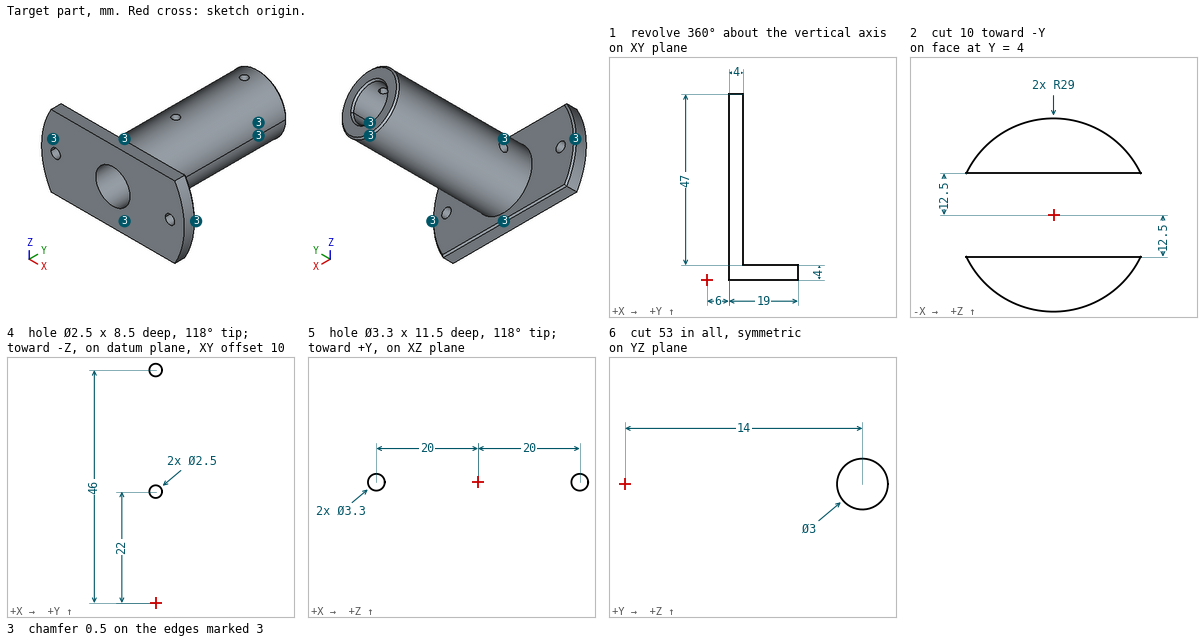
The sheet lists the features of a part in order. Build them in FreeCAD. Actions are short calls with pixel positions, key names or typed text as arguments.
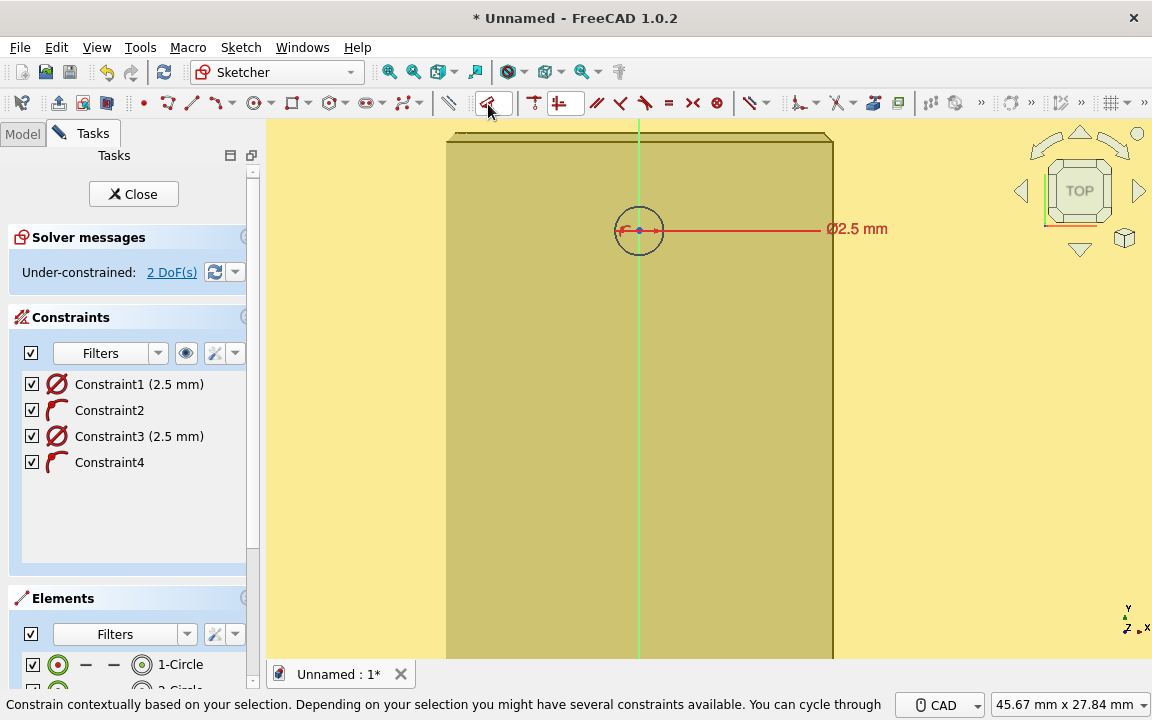
scroll(641, 229, down, 5)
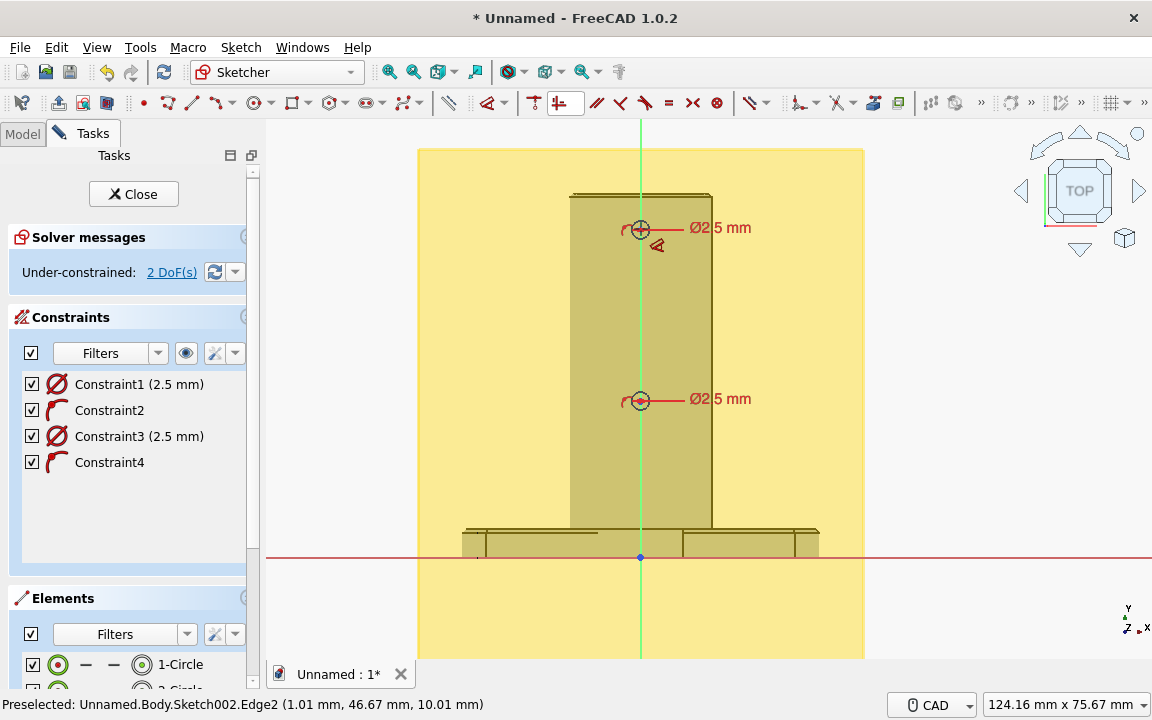
click(641, 401)
click(675, 479)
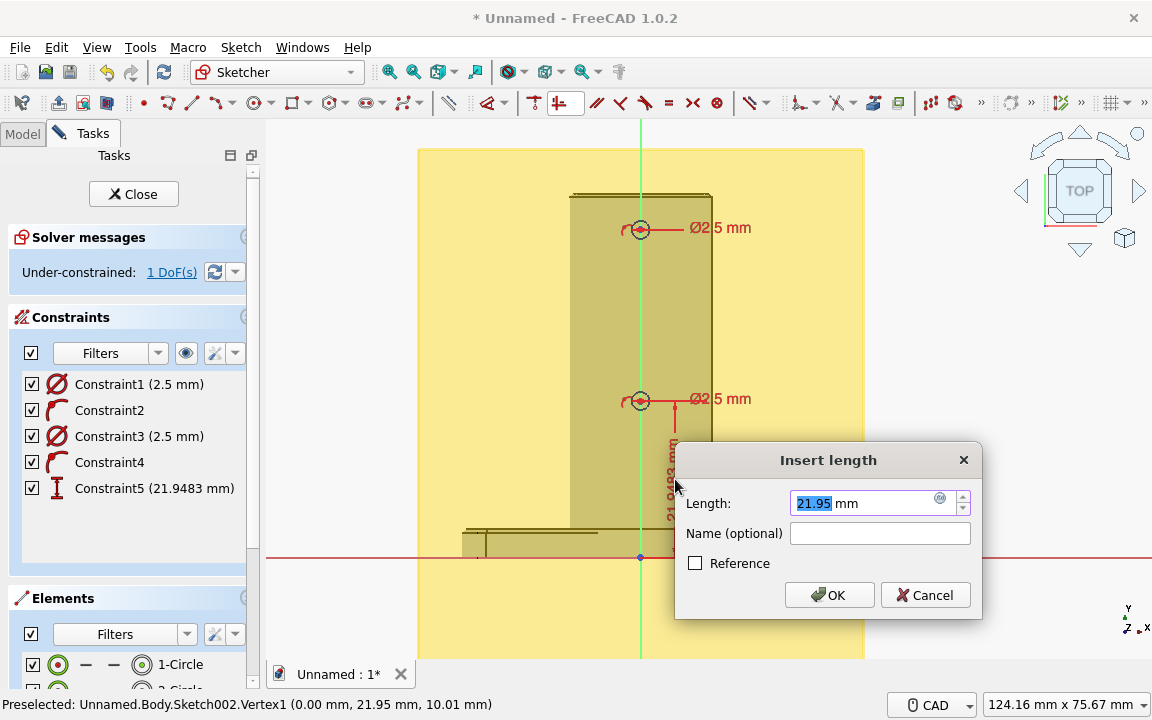
text(22)
key(Return)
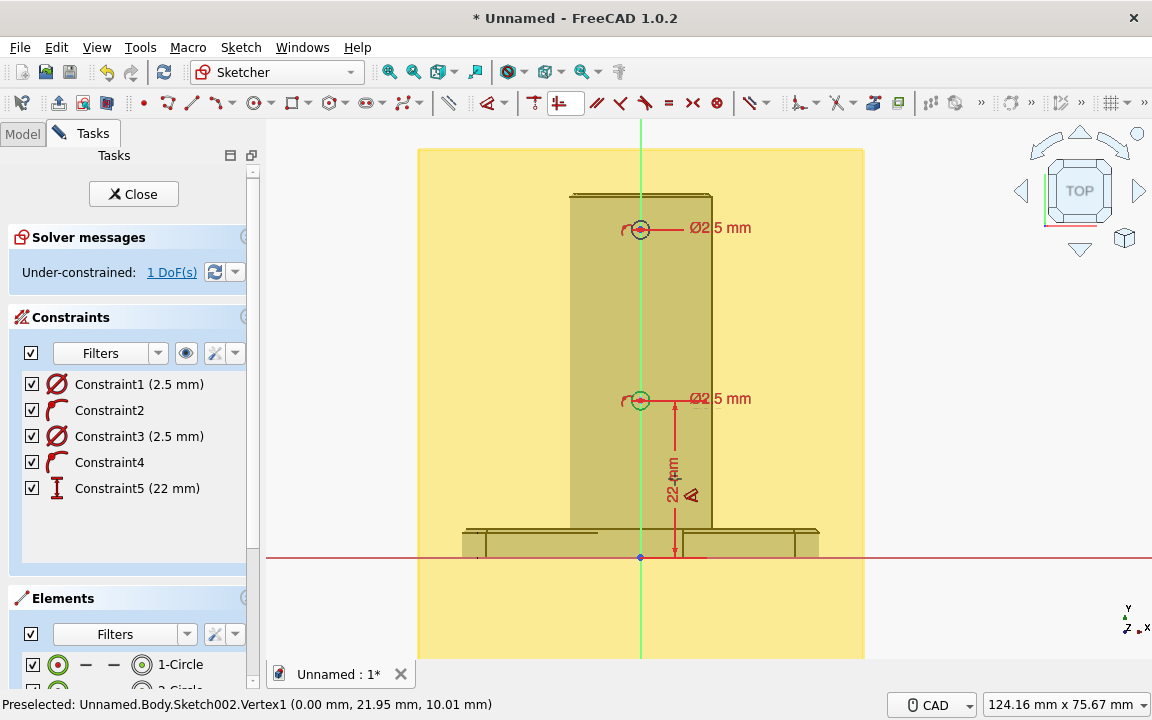
click(641, 230)
click(675, 394)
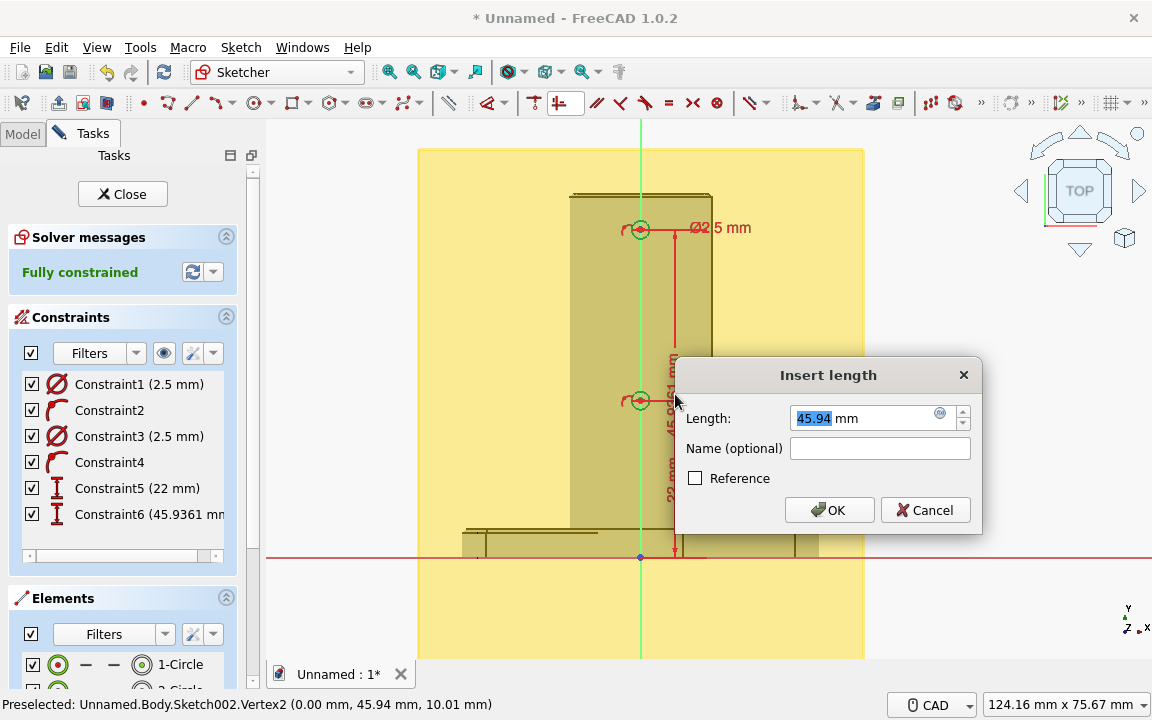
text(46)
key(Return)
key(Escape)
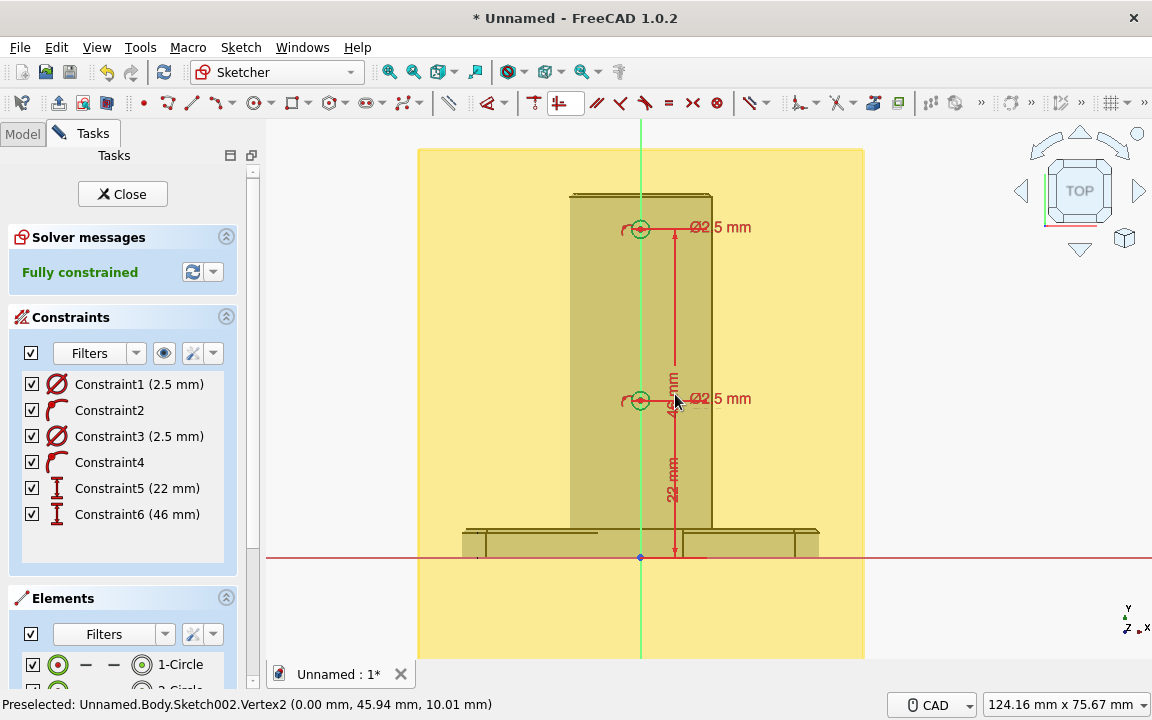
click(123, 194)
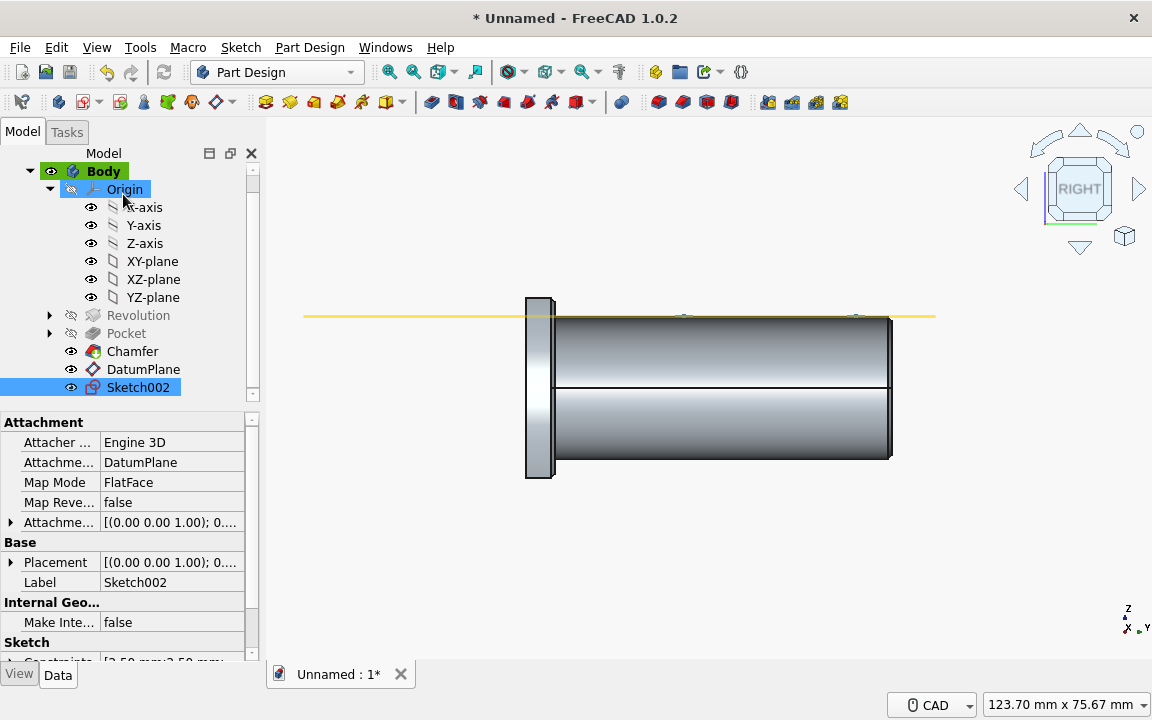
click(456, 102)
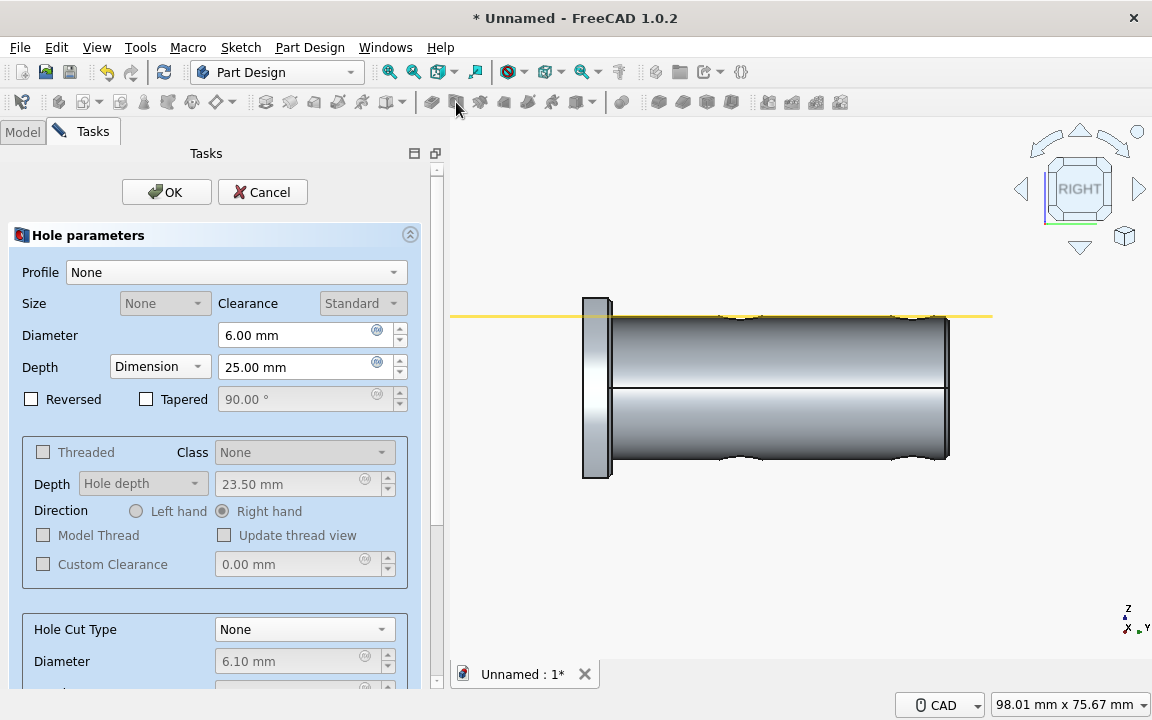
triple_click(305, 335)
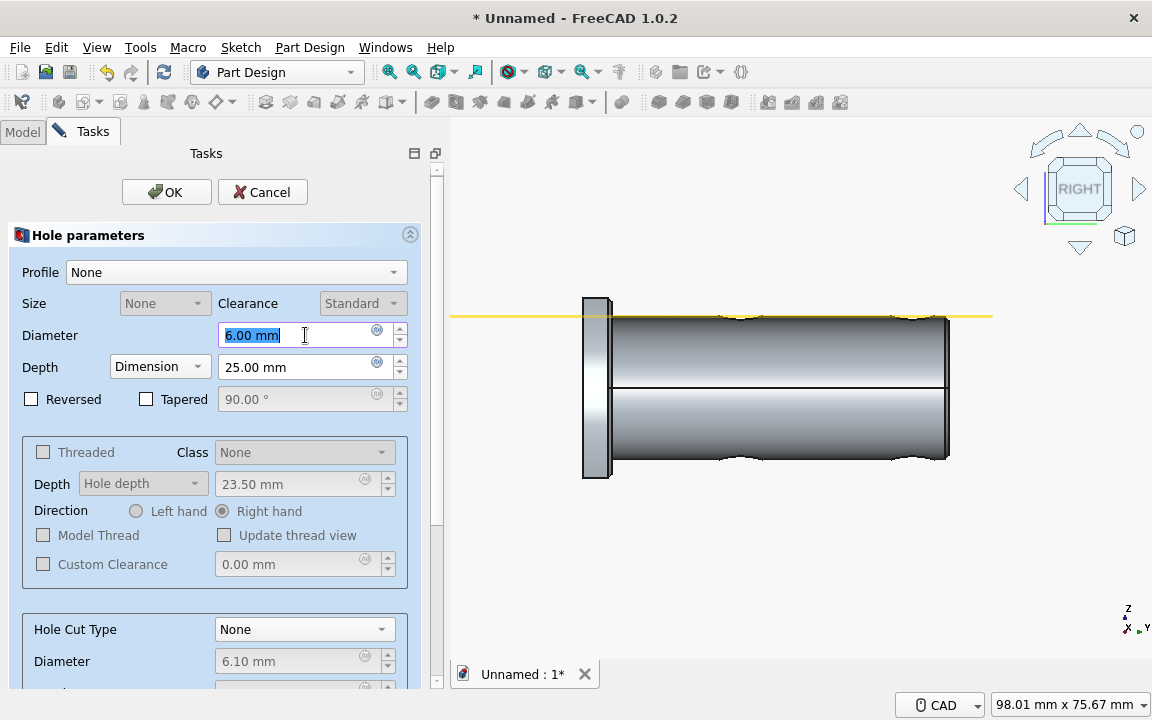
text(2.5)
key(Tab)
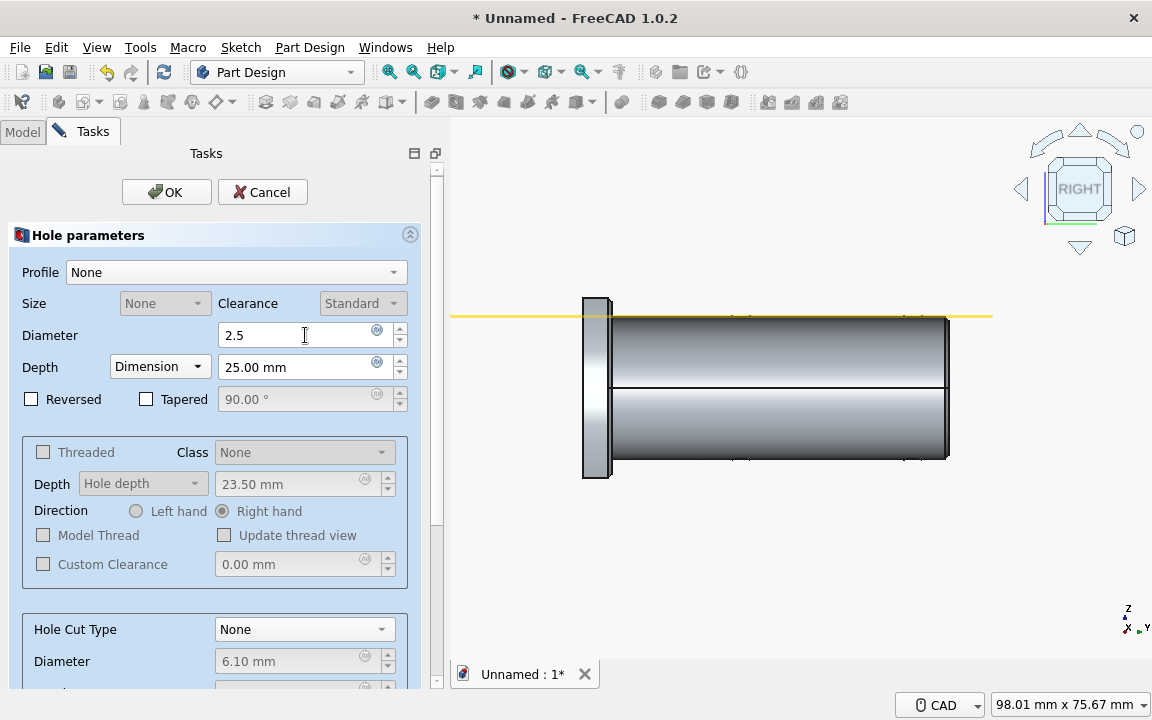
triple_click(305, 367)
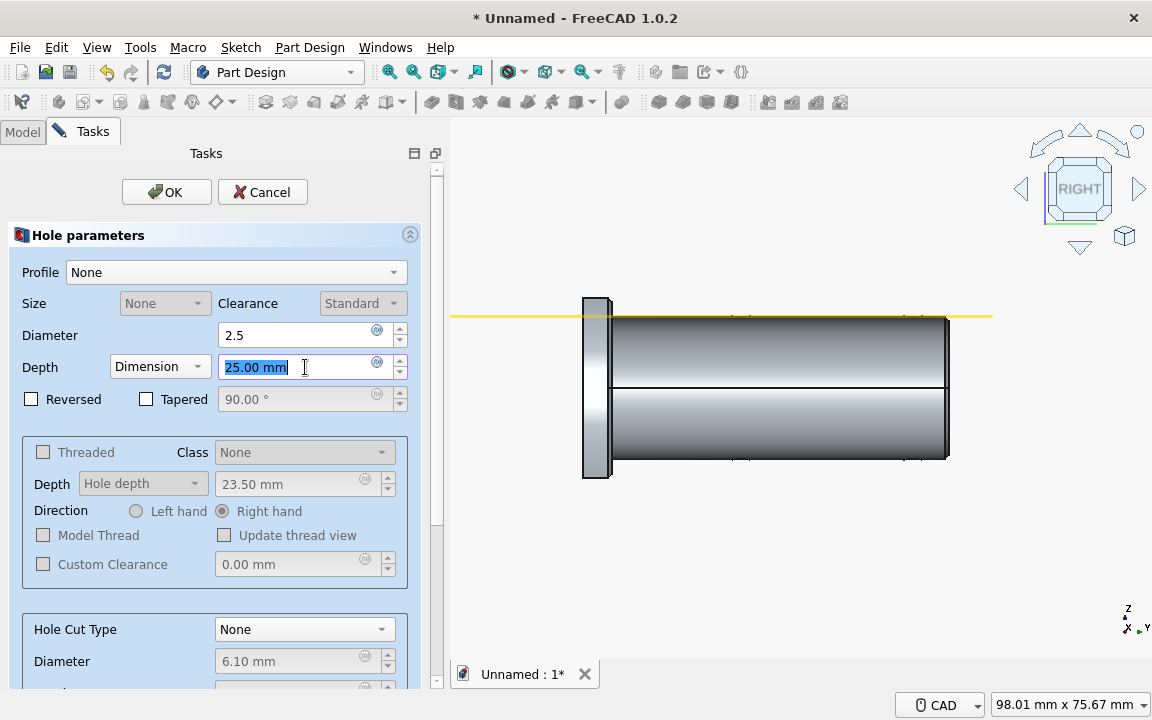
text(8.5)
key(Tab)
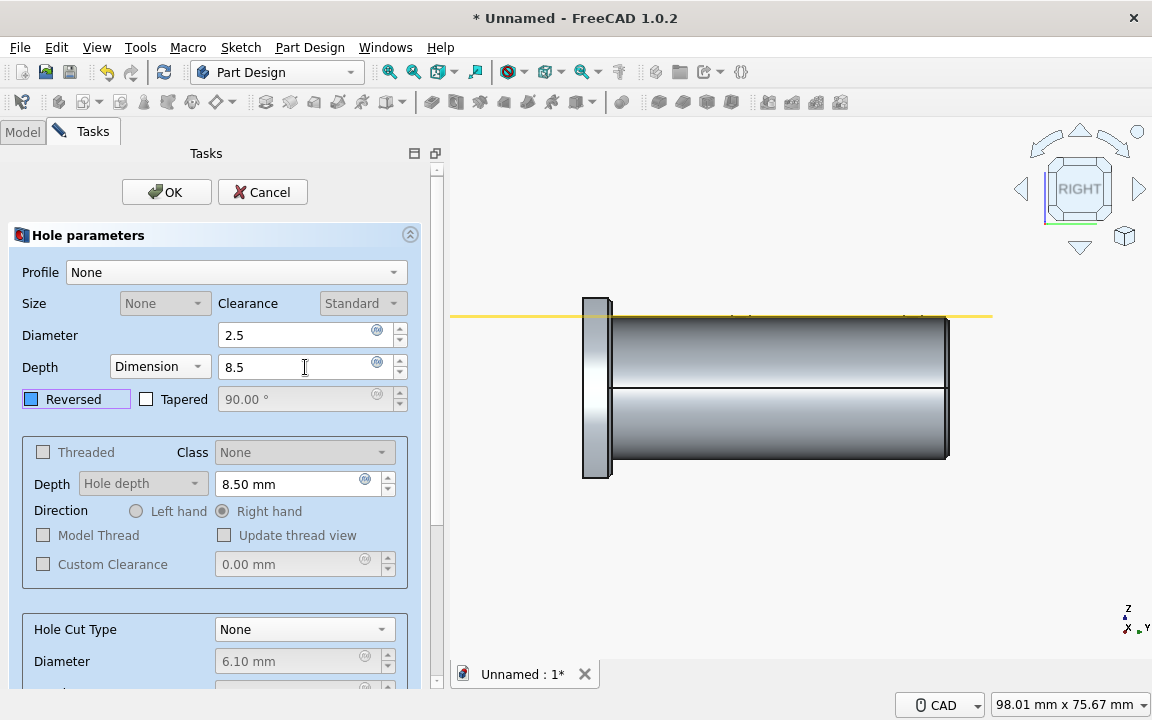
click(167, 192)